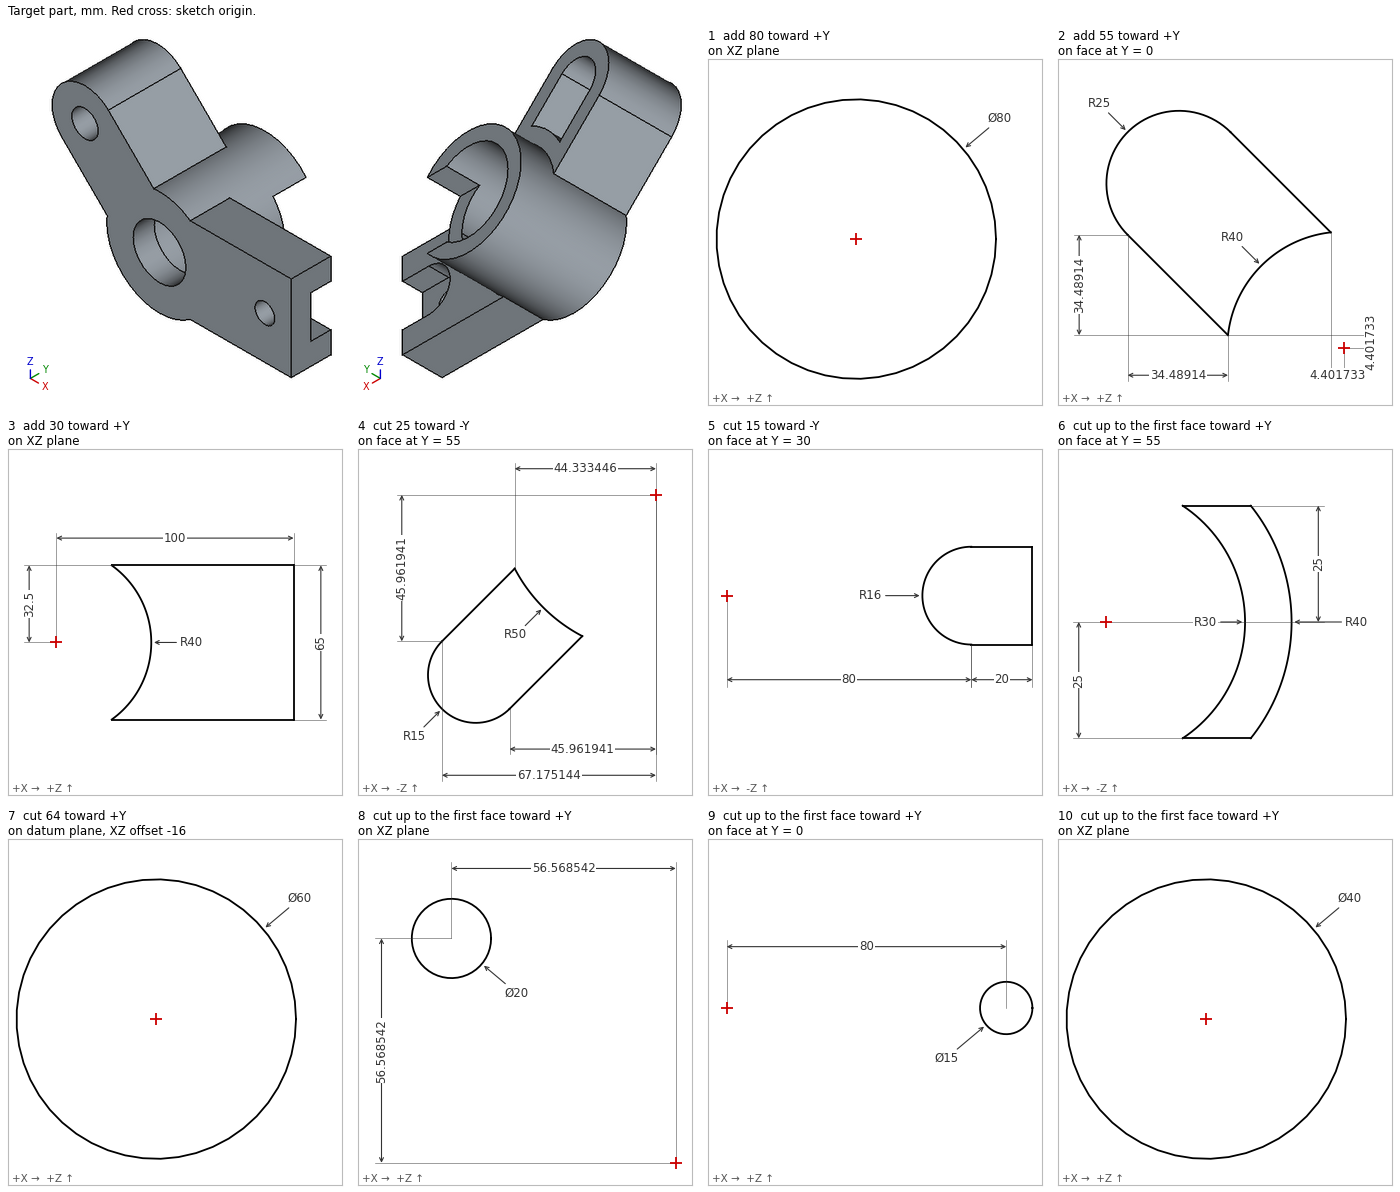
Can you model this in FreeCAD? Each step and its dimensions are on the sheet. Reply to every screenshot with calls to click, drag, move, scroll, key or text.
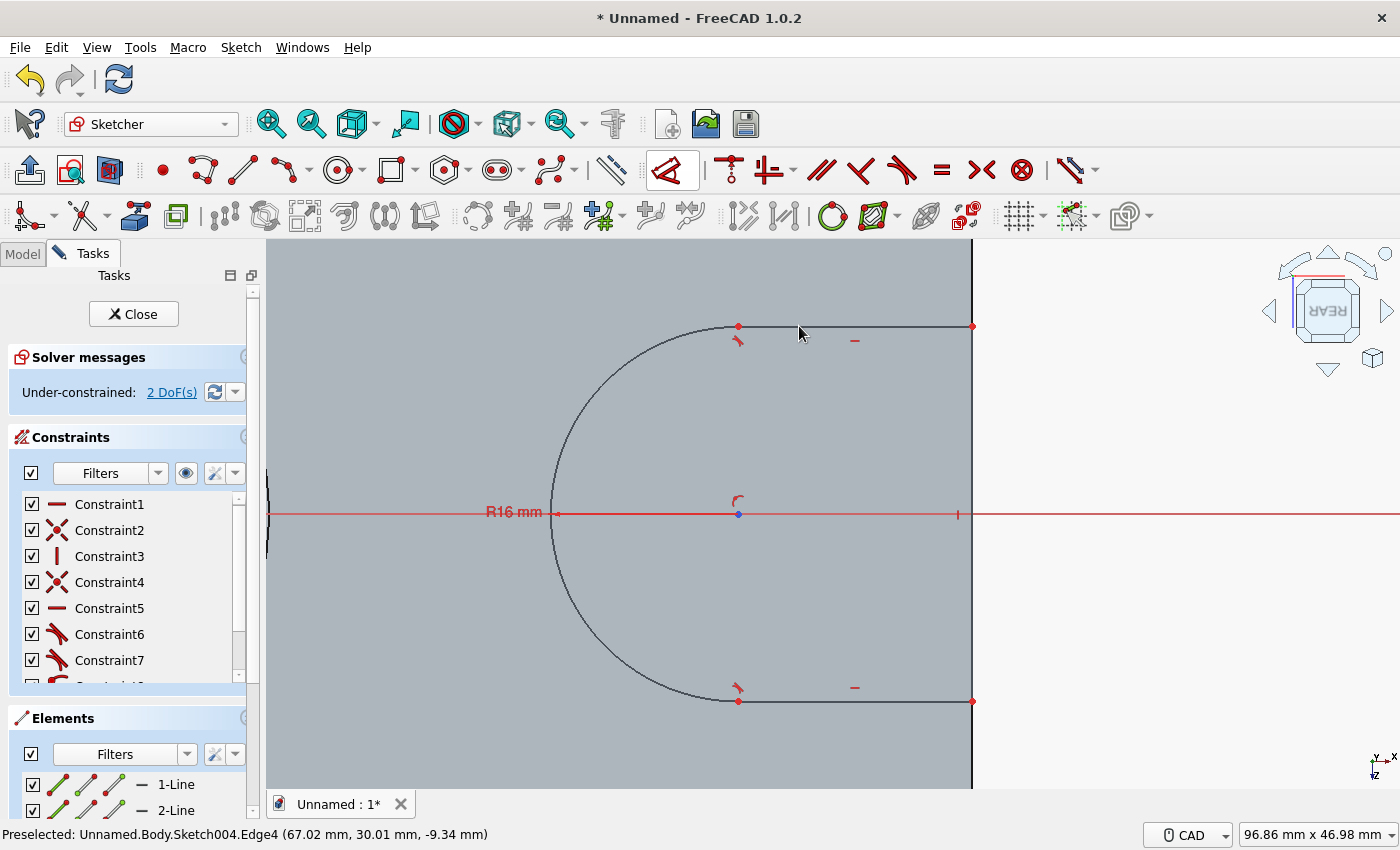
click(808, 702)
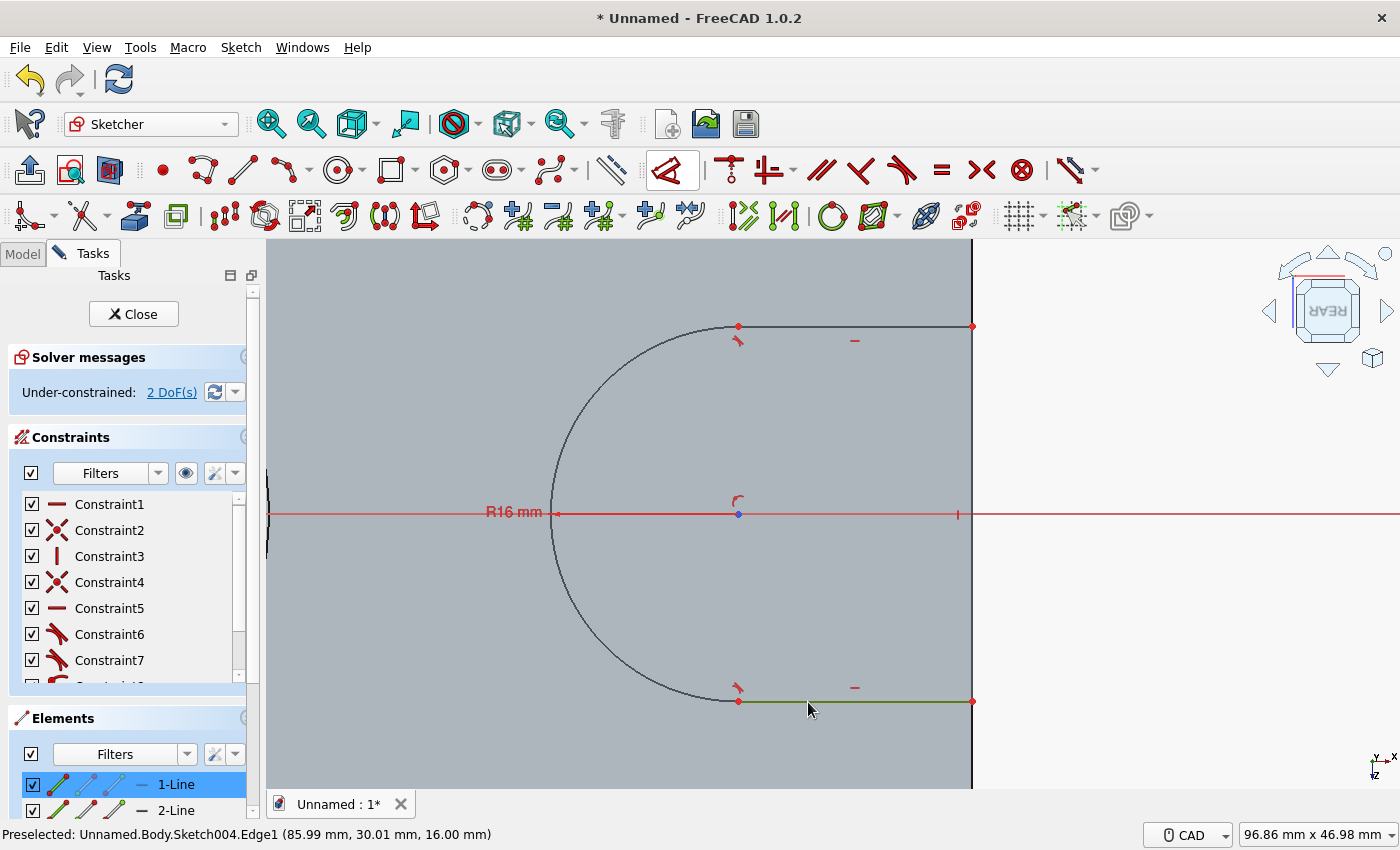
click(694, 170)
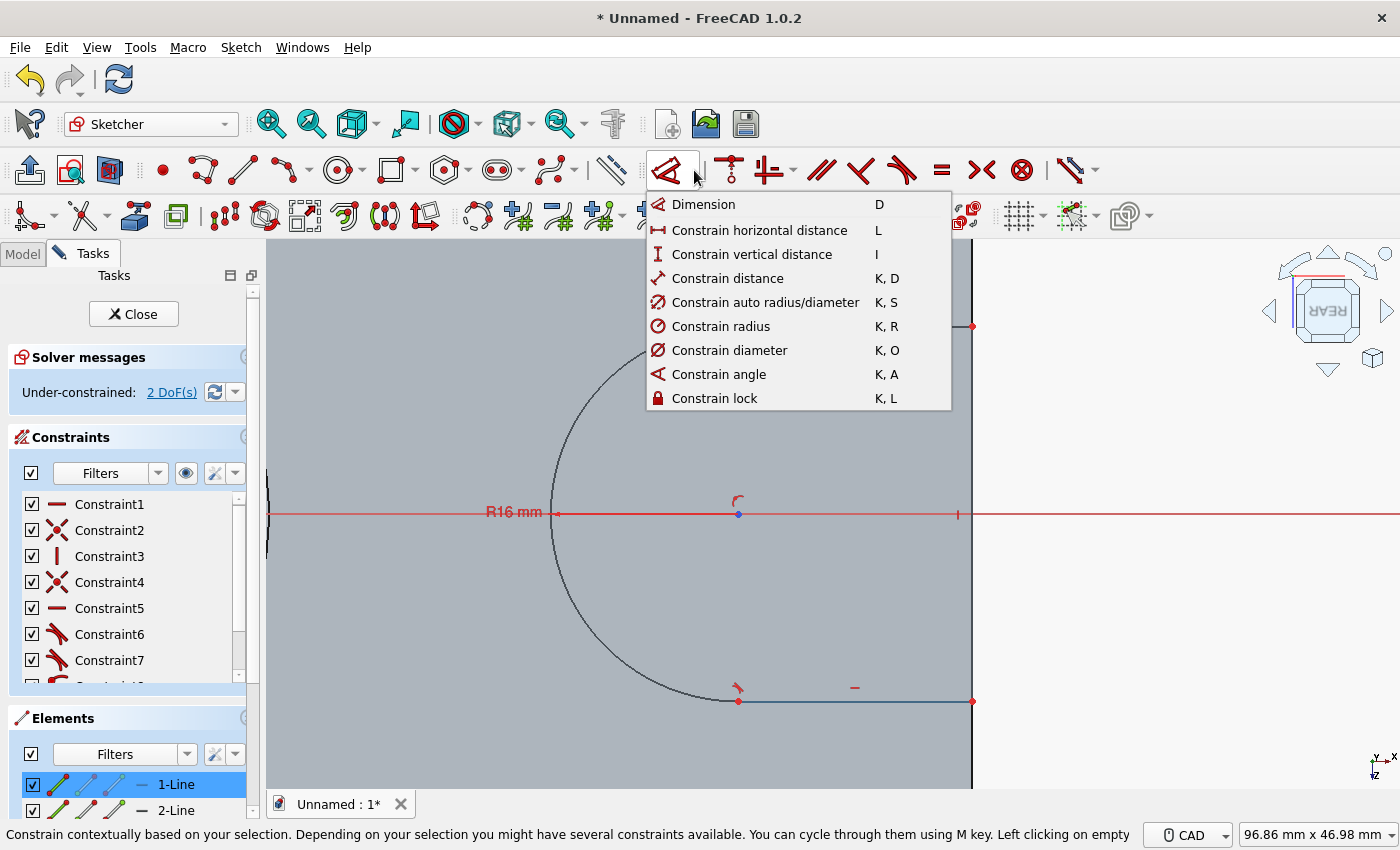
click(799, 230)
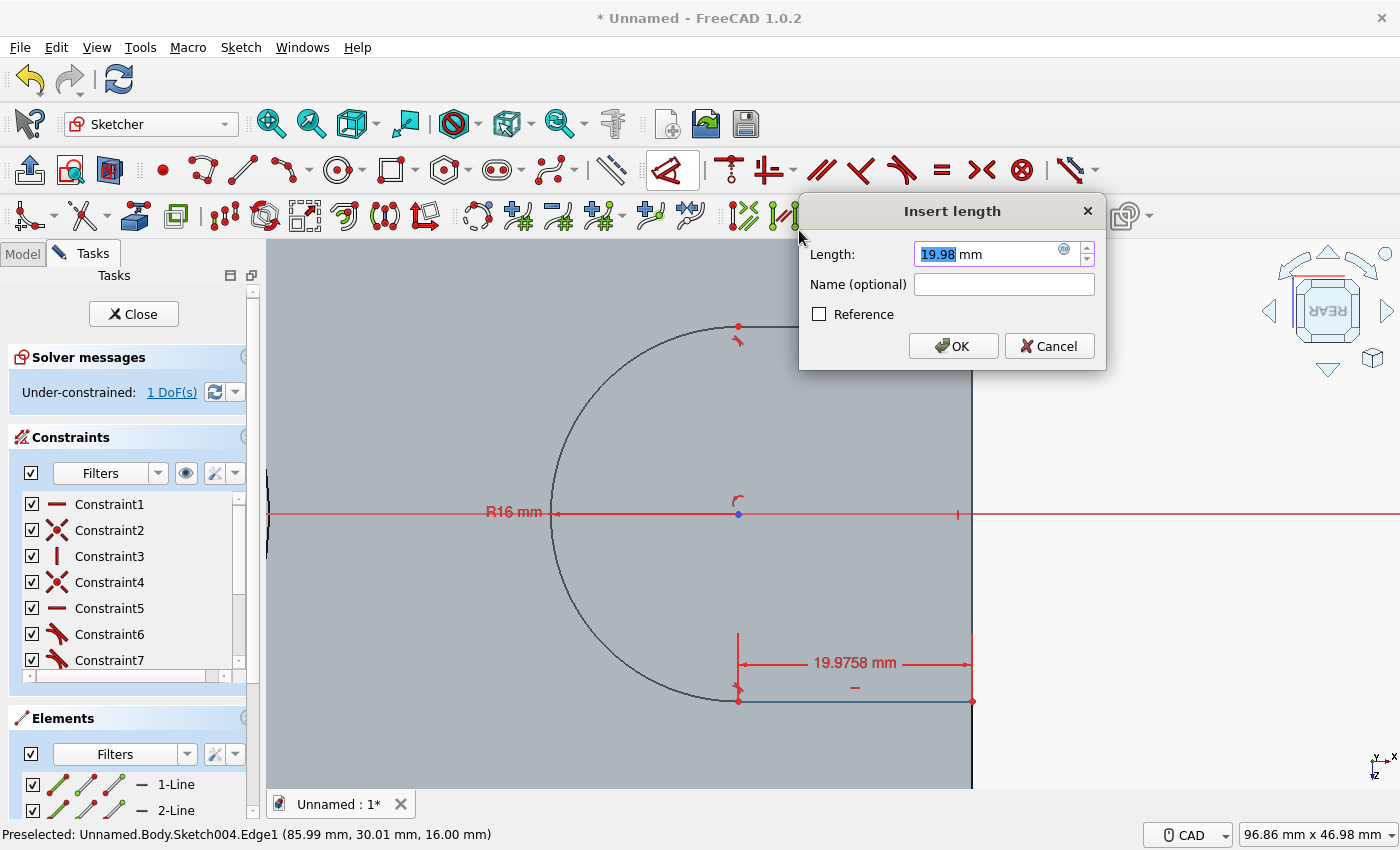
text(20)
key(Return)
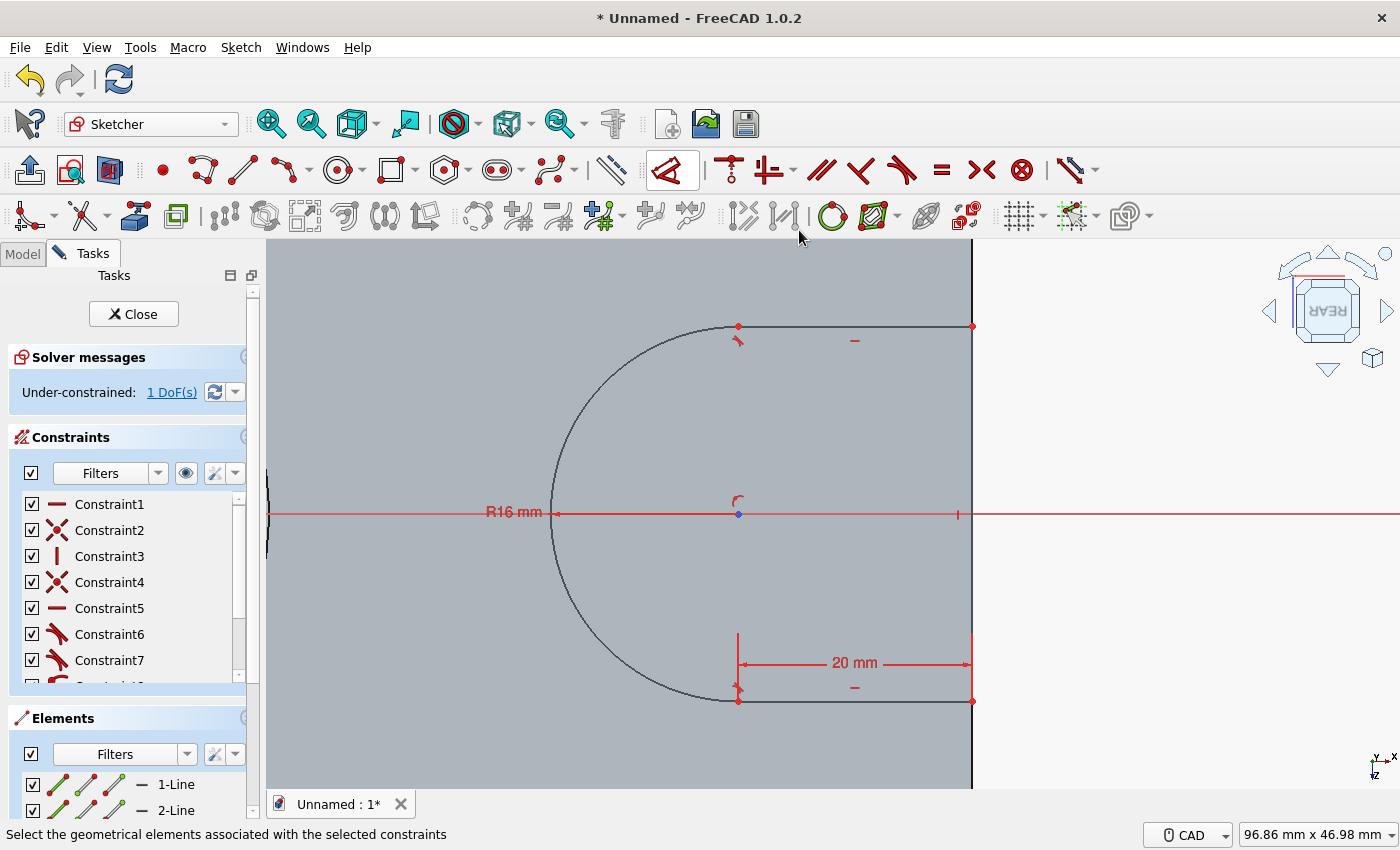
click(738, 702)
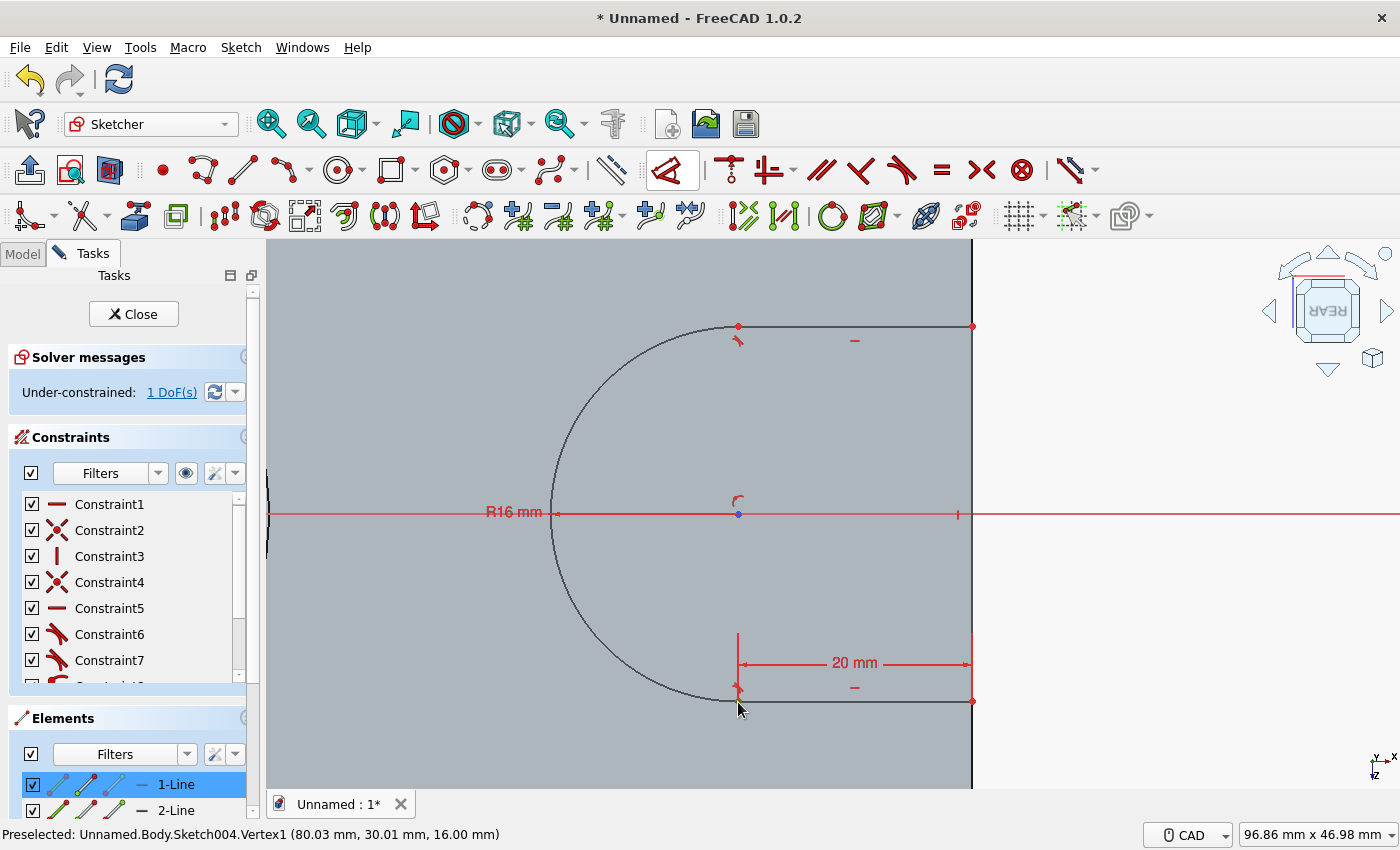
click(694, 170)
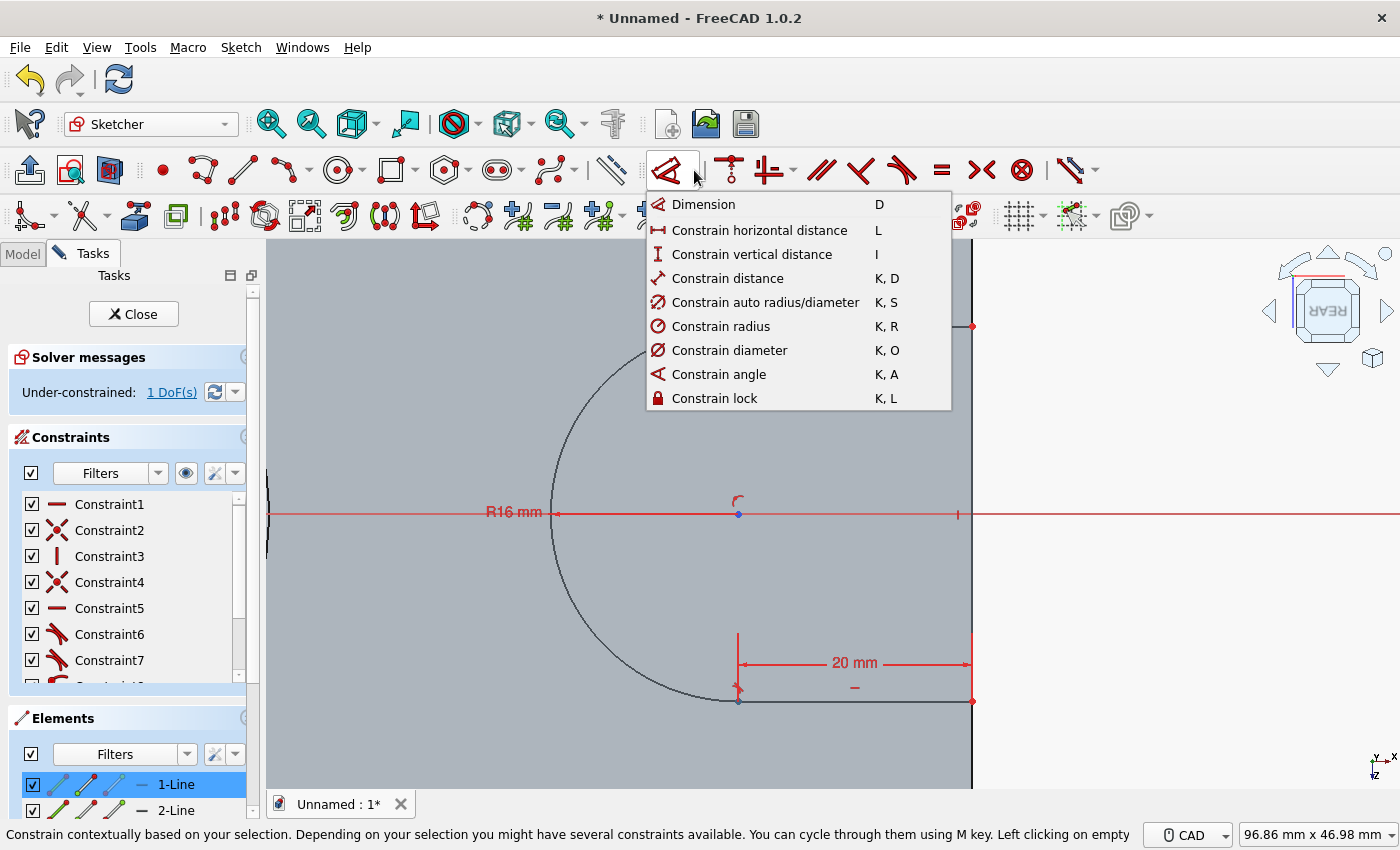
click(799, 230)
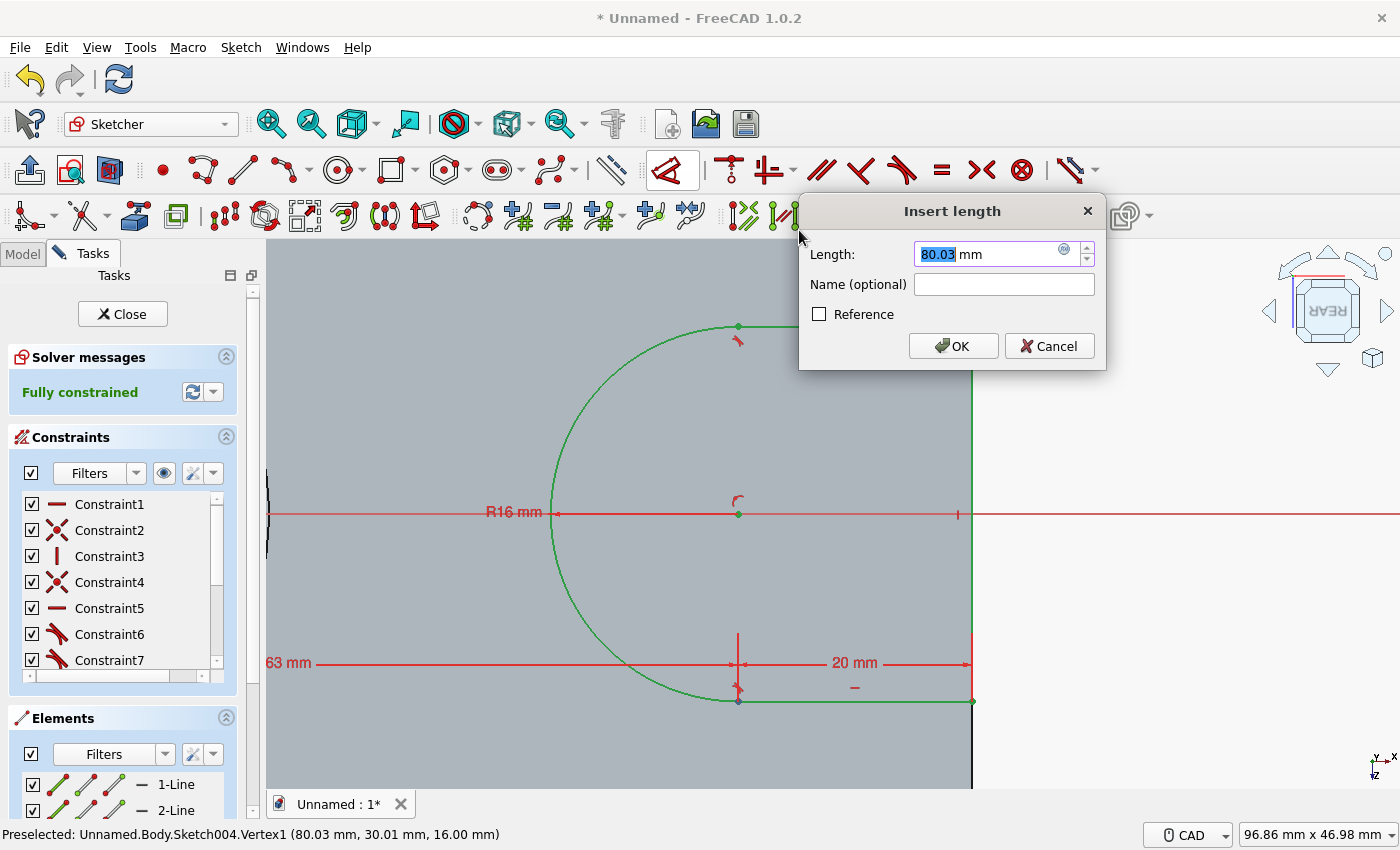
text(80)
key(Return)